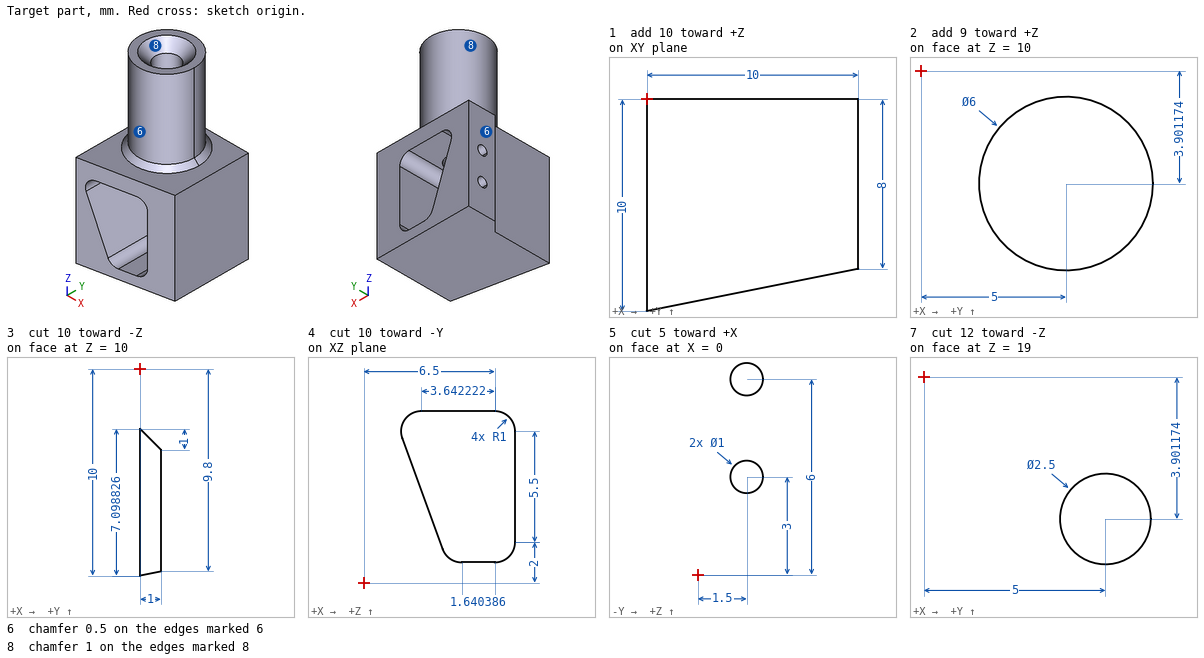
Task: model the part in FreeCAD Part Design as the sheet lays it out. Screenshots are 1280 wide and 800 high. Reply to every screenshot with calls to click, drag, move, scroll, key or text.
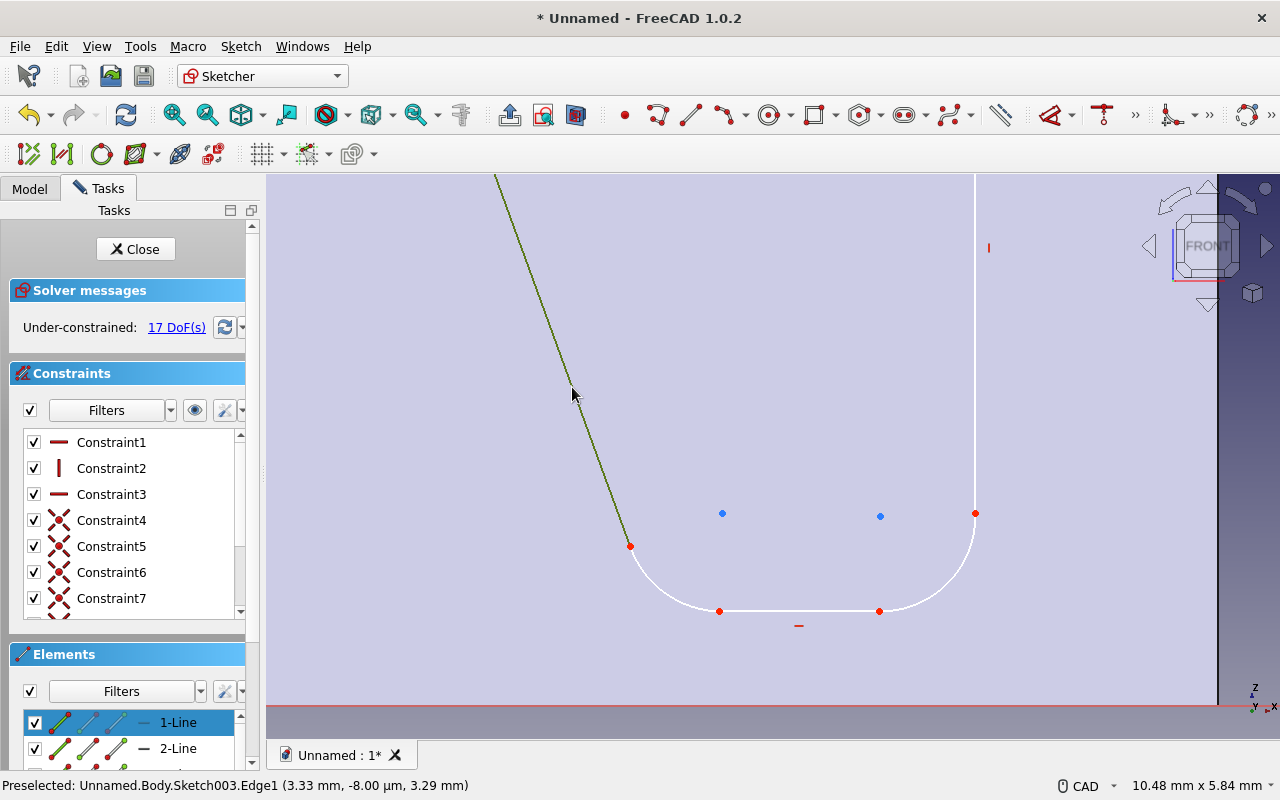
scroll(779, 589, down, 4)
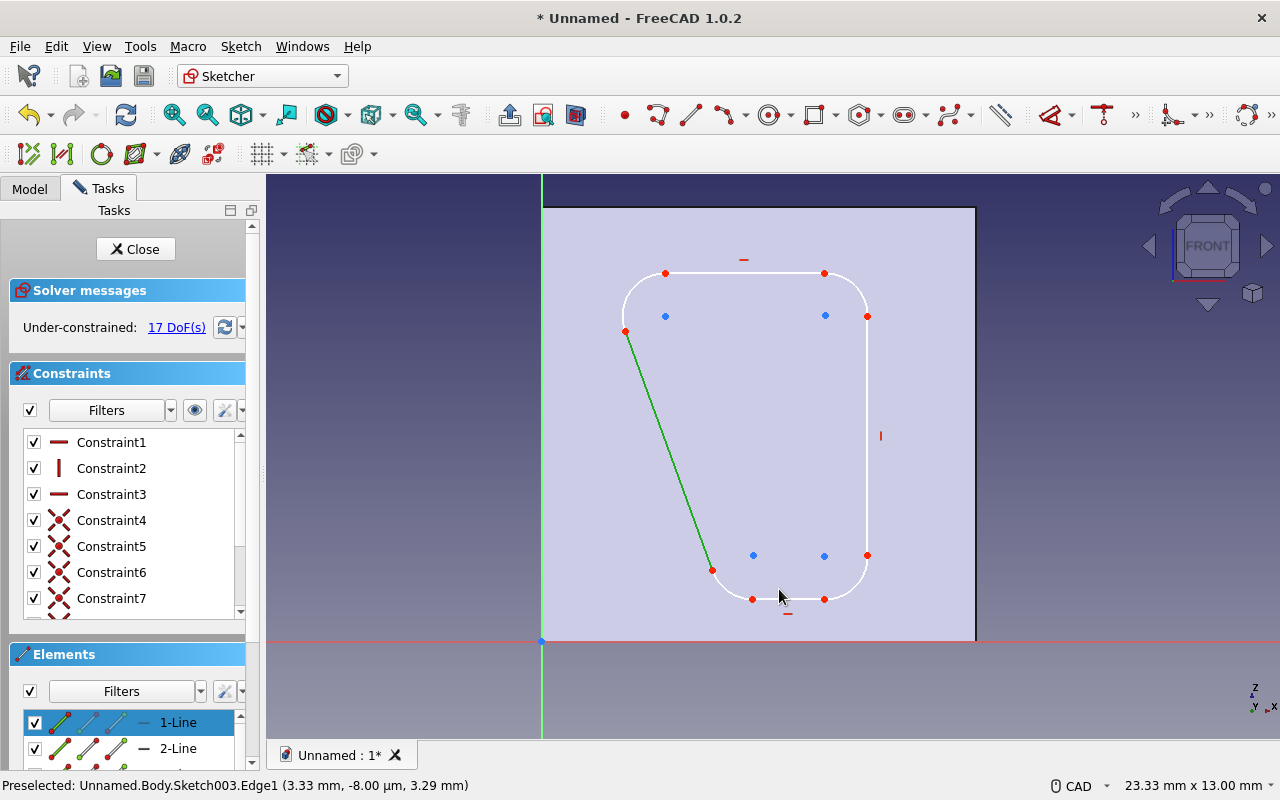
click(642, 280)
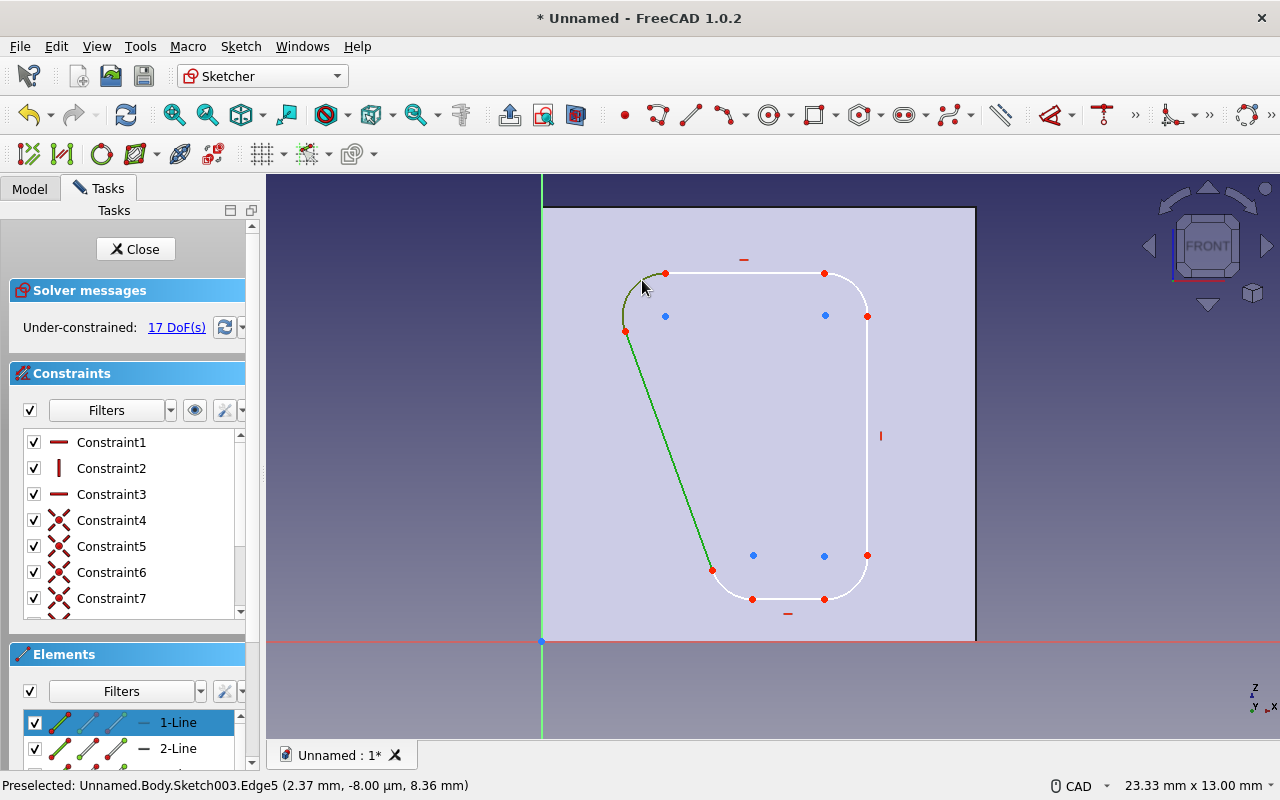
key(t)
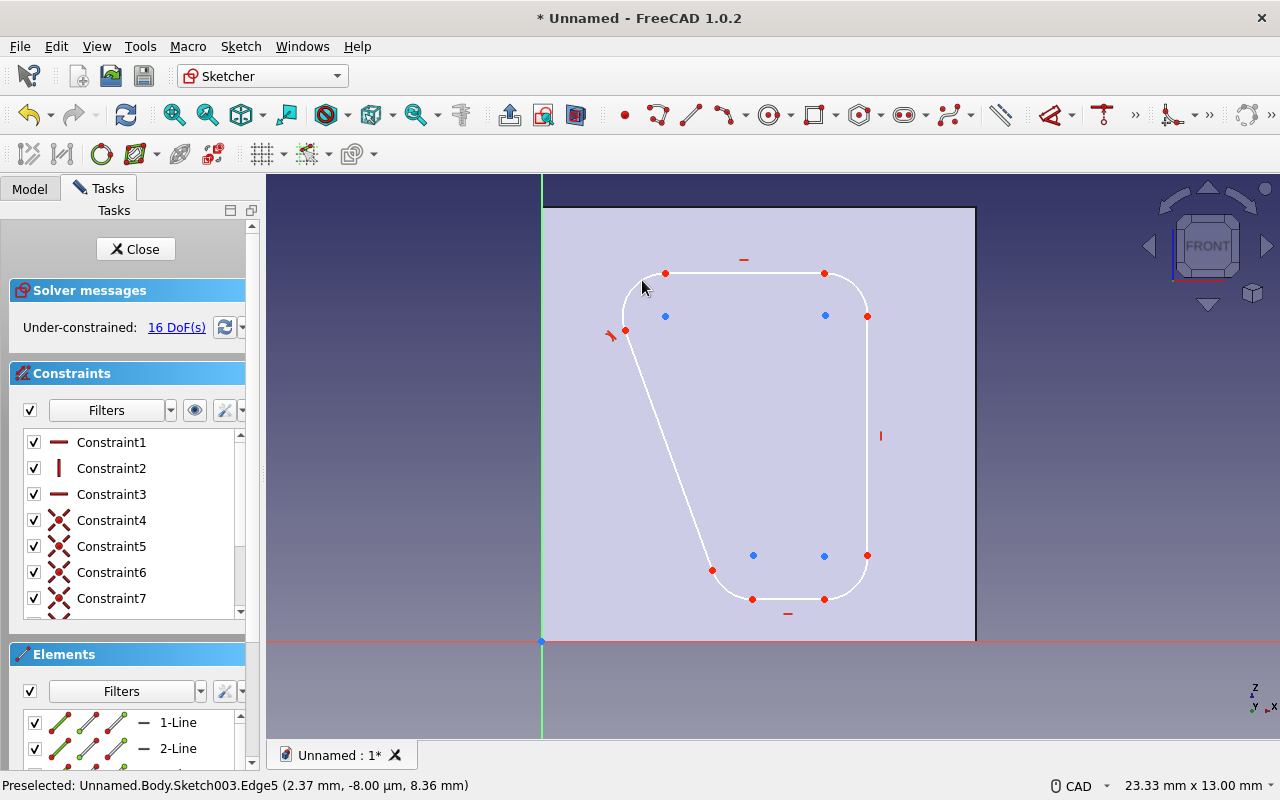
click(686, 499)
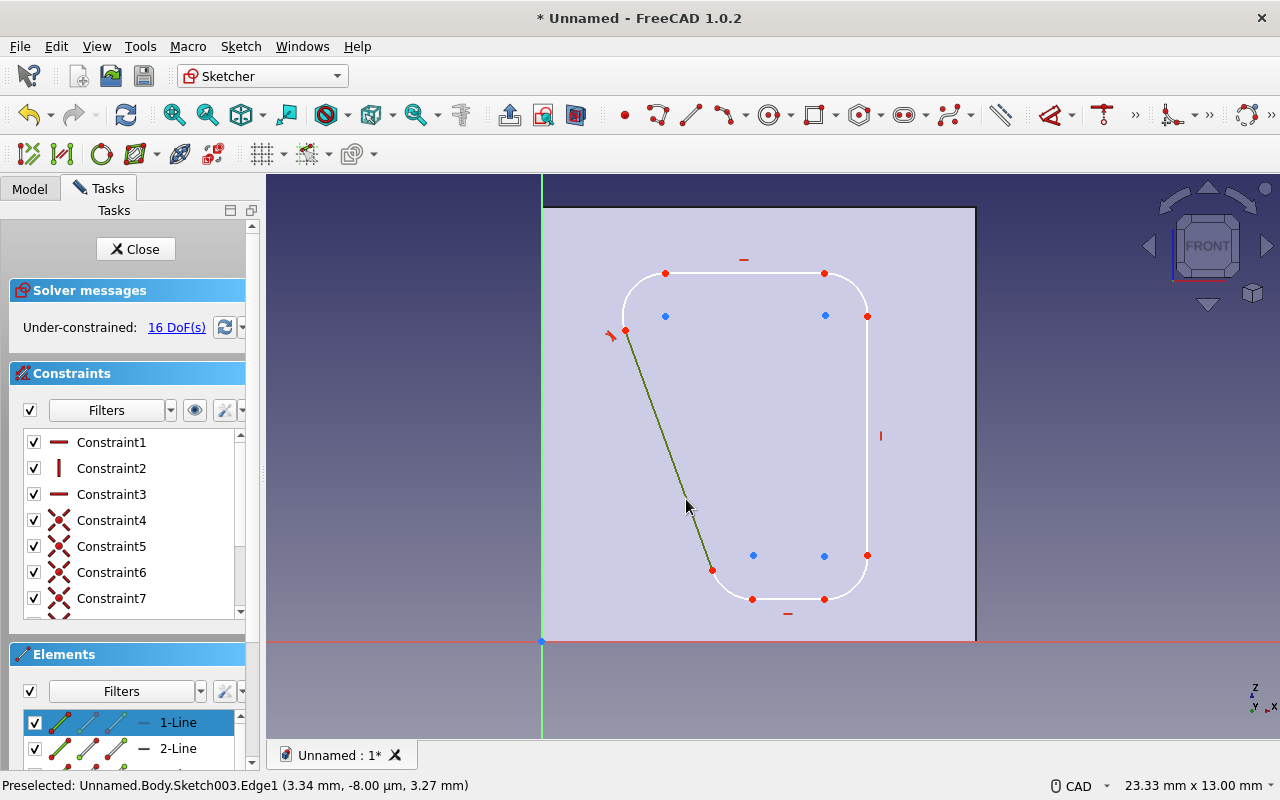
click(720, 584)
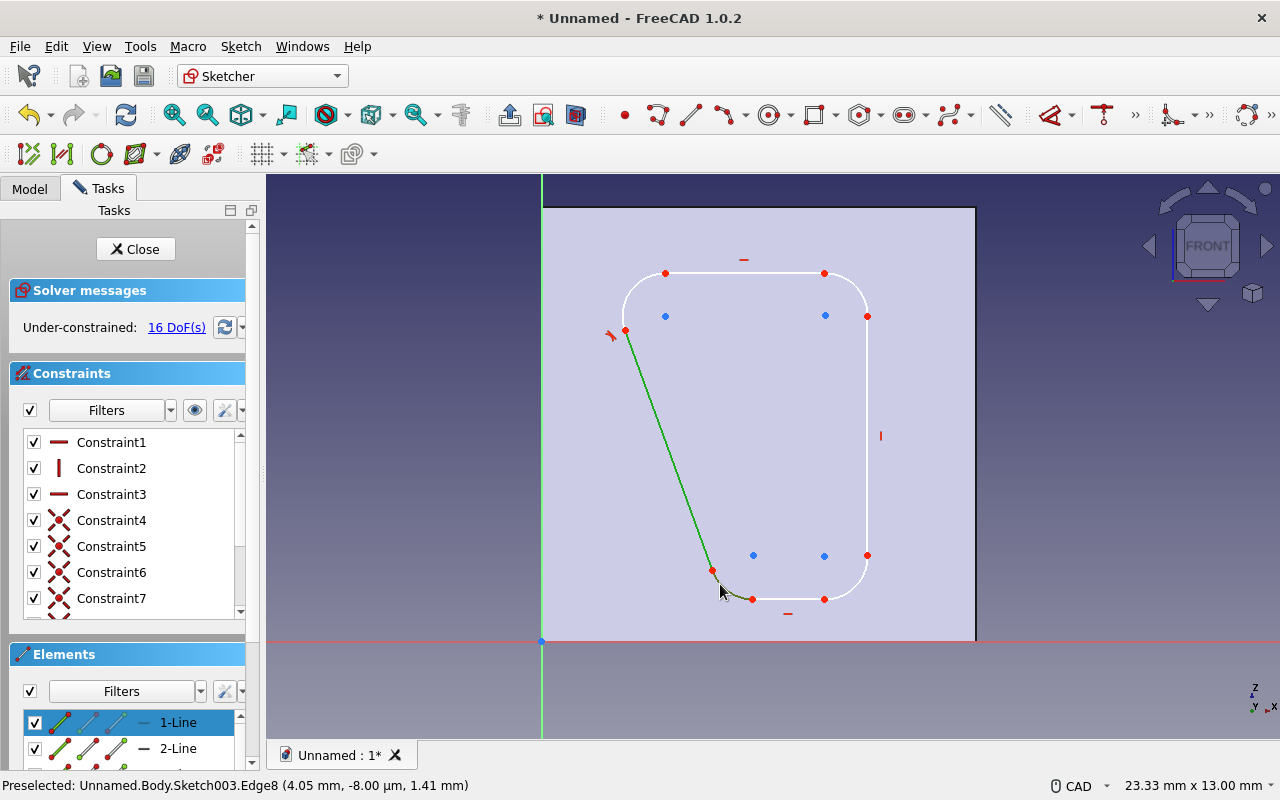
key(t)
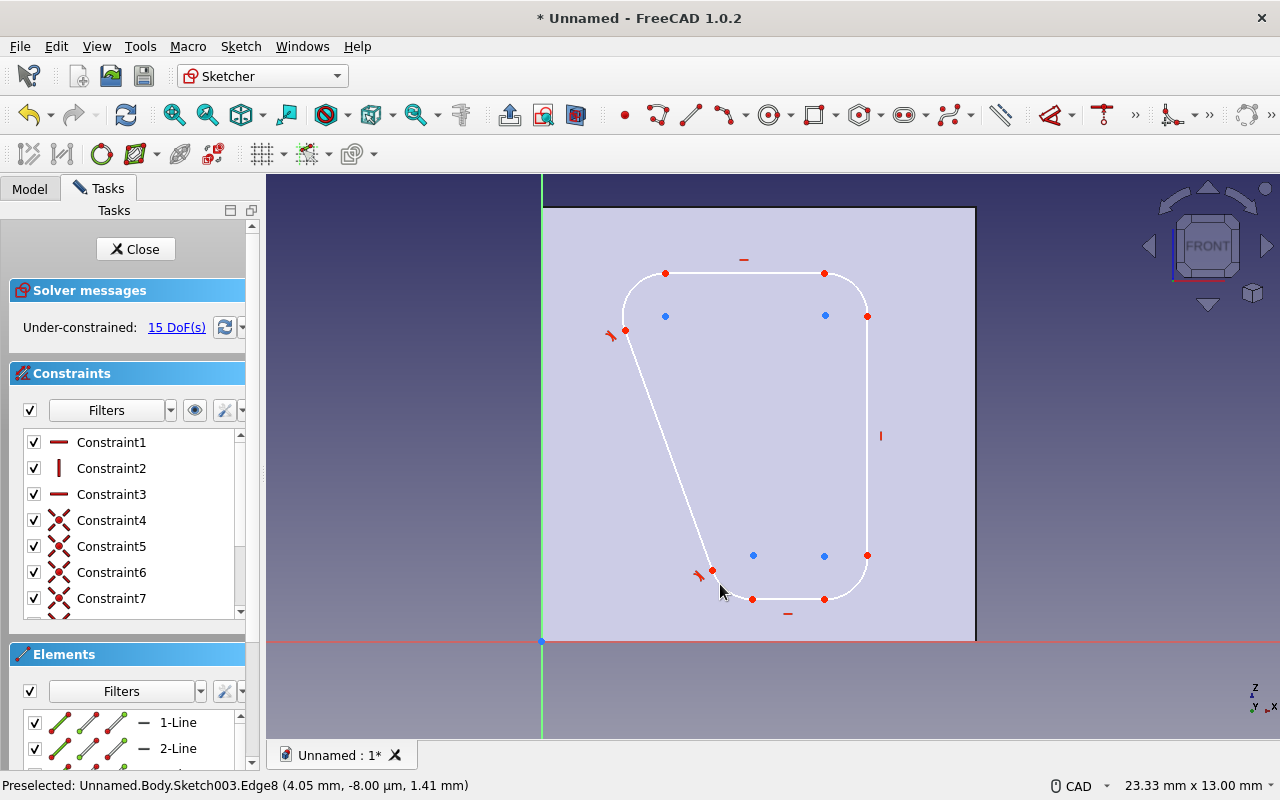
click(713, 273)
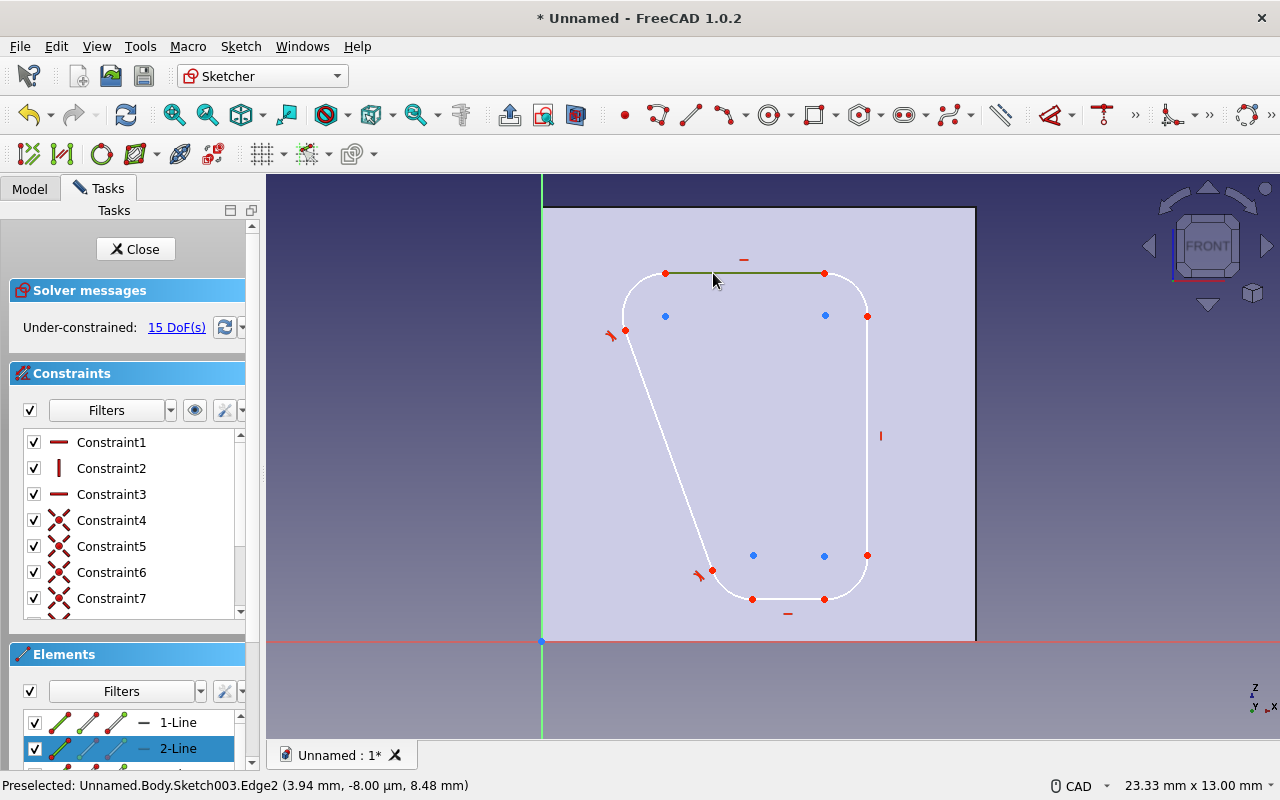
click(642, 280)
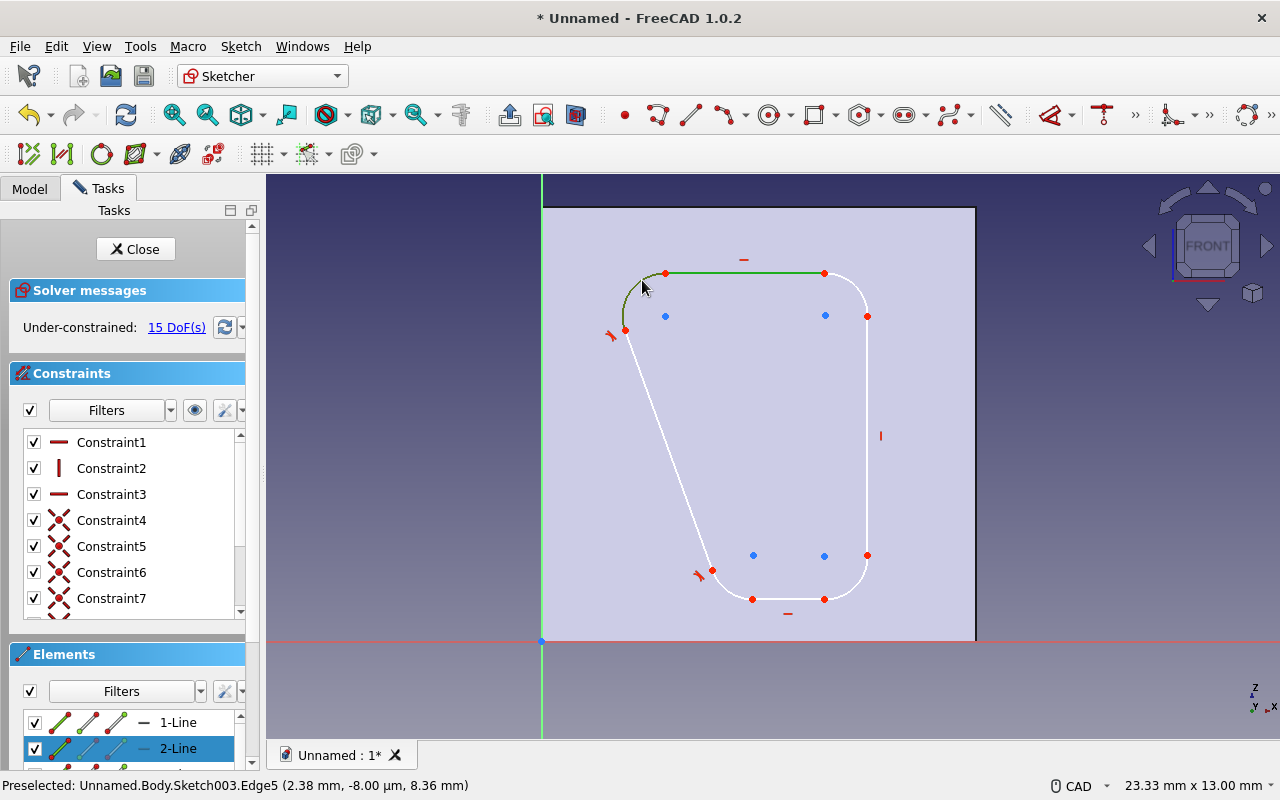
key(t)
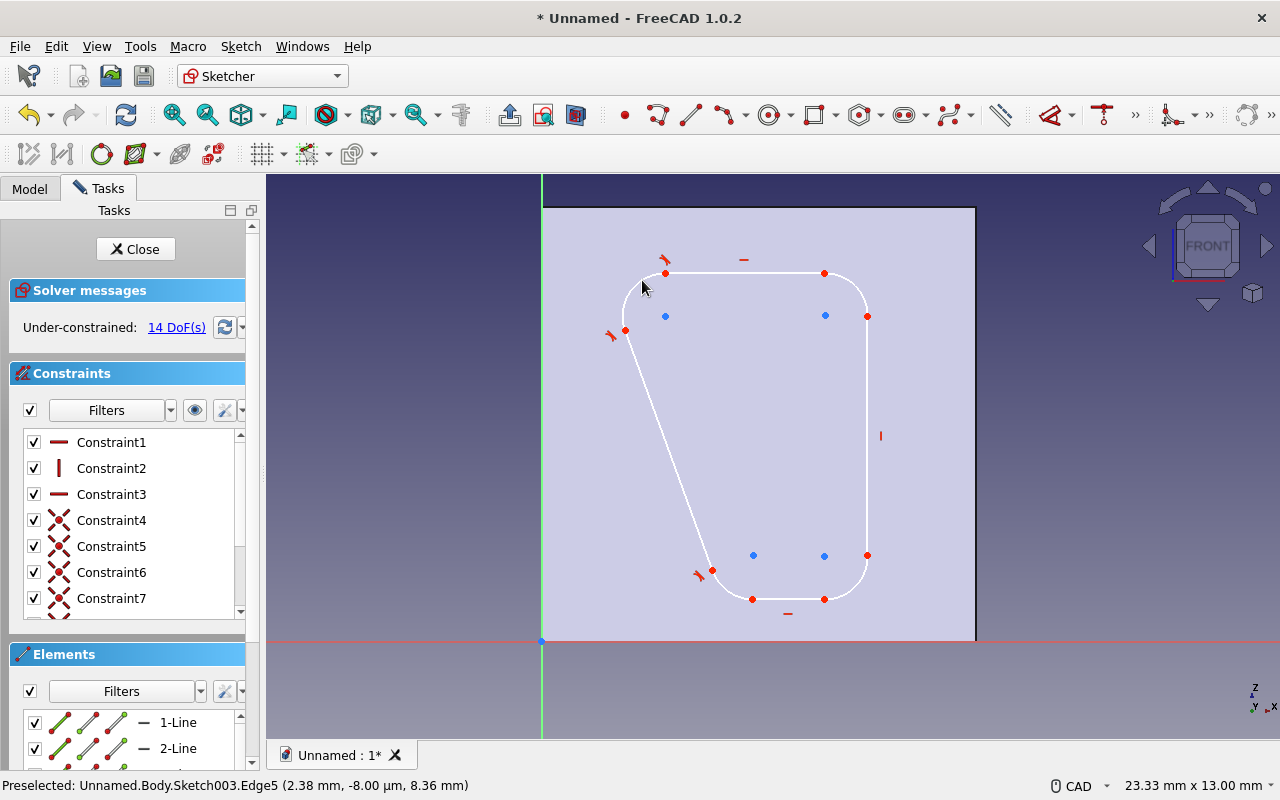
click(713, 273)